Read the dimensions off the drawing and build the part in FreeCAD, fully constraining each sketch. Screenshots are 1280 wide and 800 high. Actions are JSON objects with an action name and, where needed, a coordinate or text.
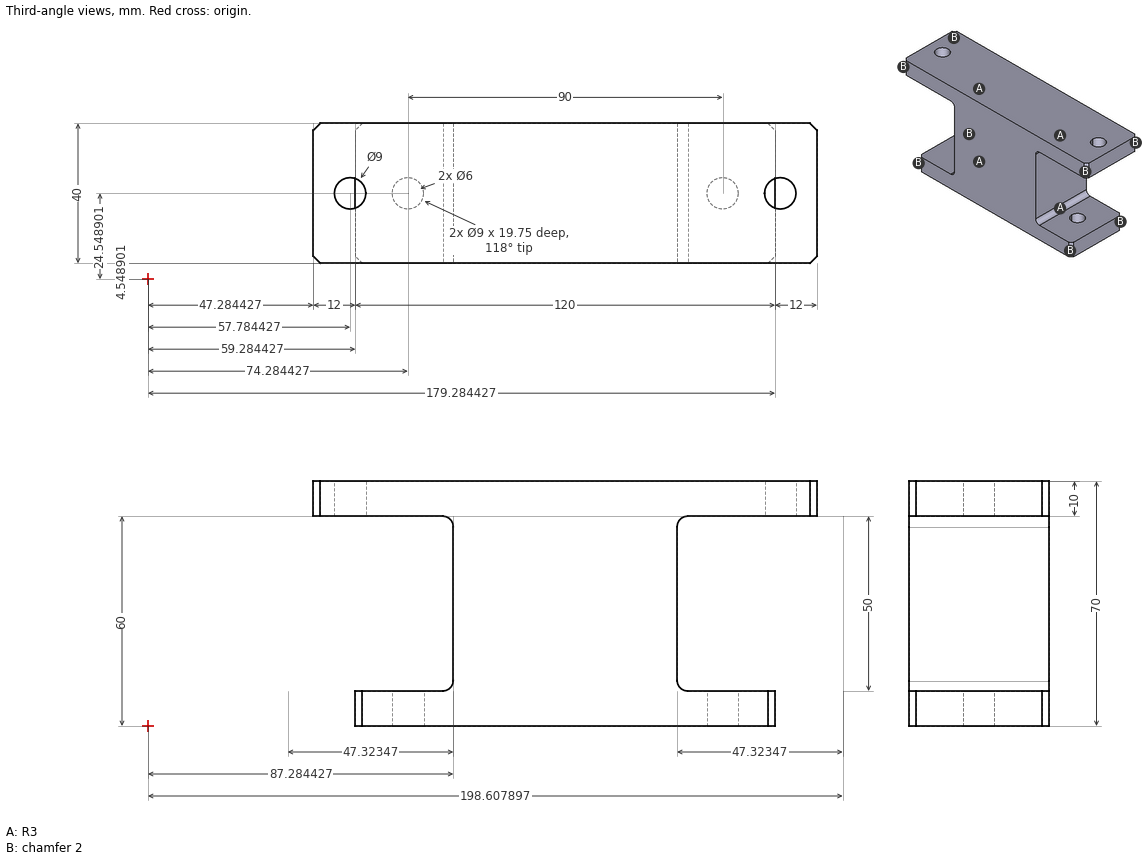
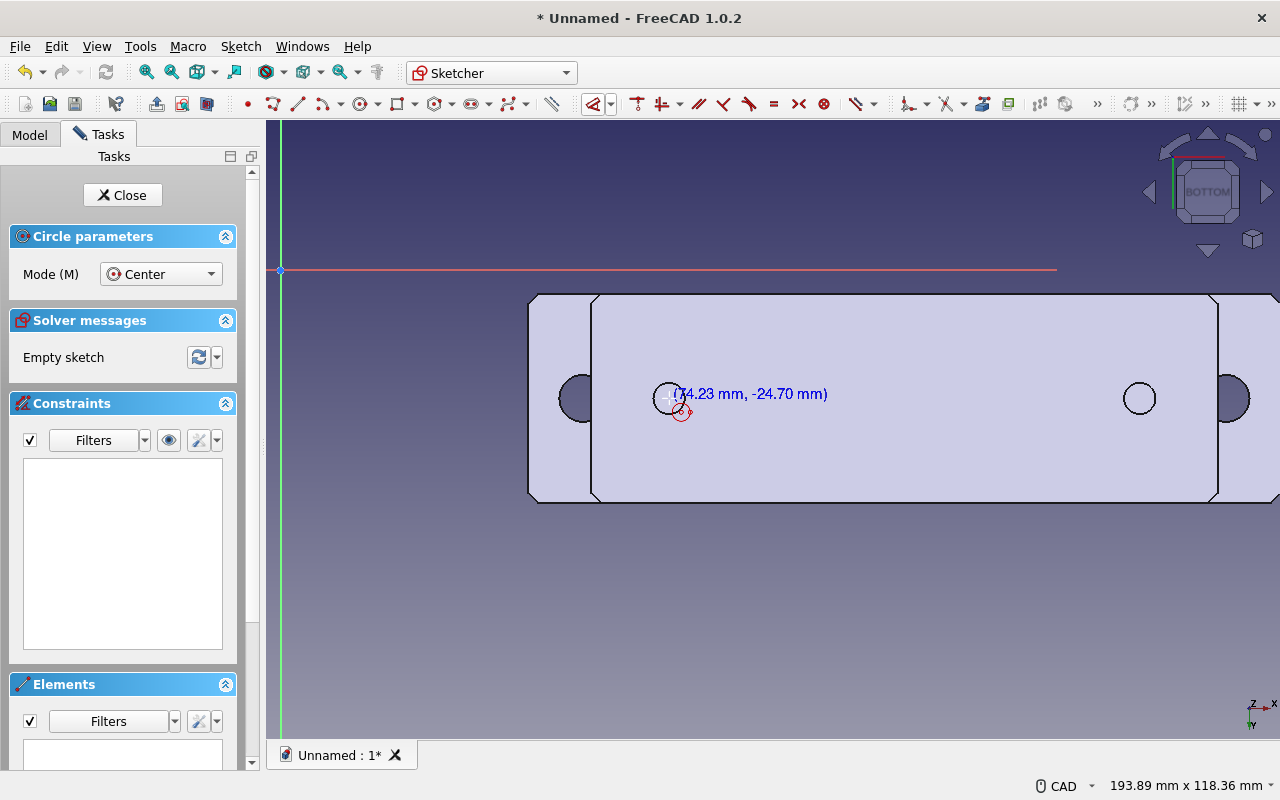
{"action": "left_click", "coordinate": [669, 398]}
{"action": "left_click", "coordinate": [686, 382]}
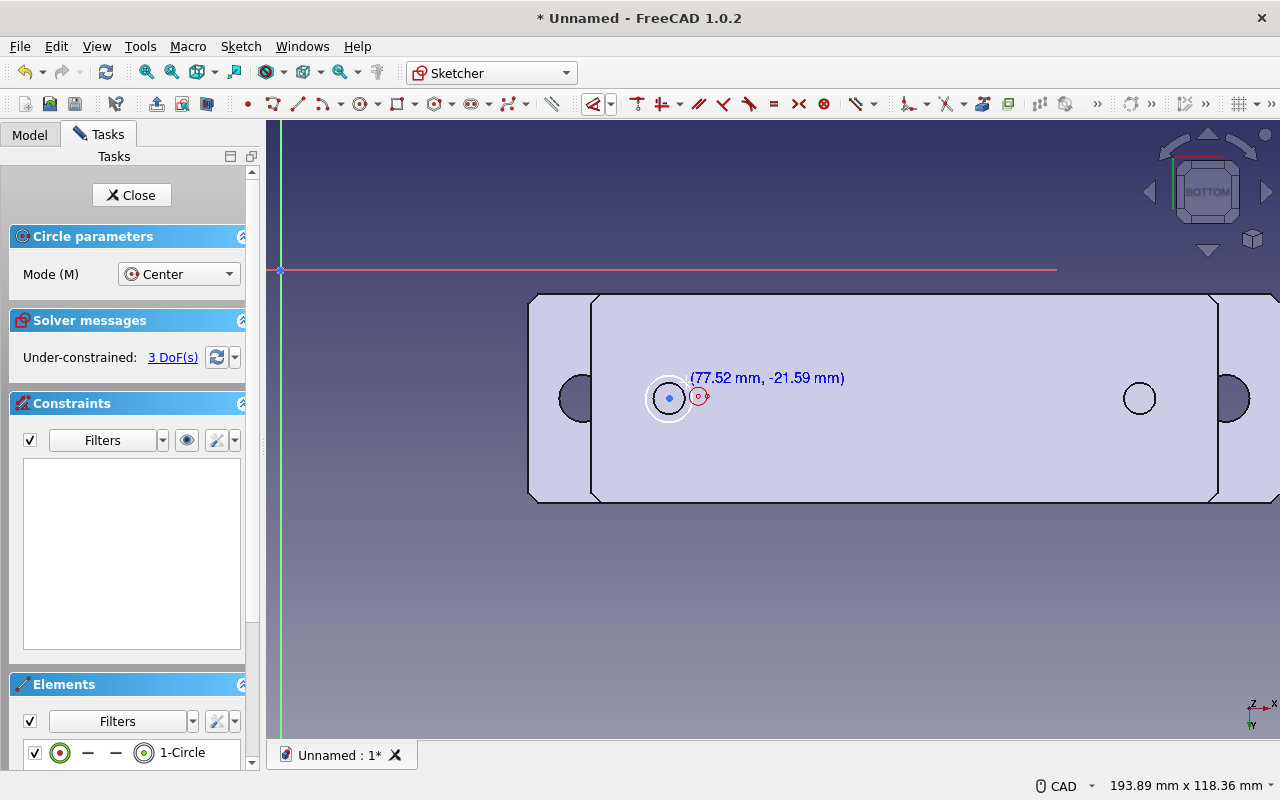
{"action": "scroll", "coordinate": [669, 599], "scroll_direction": "down", "scroll_amount": 2}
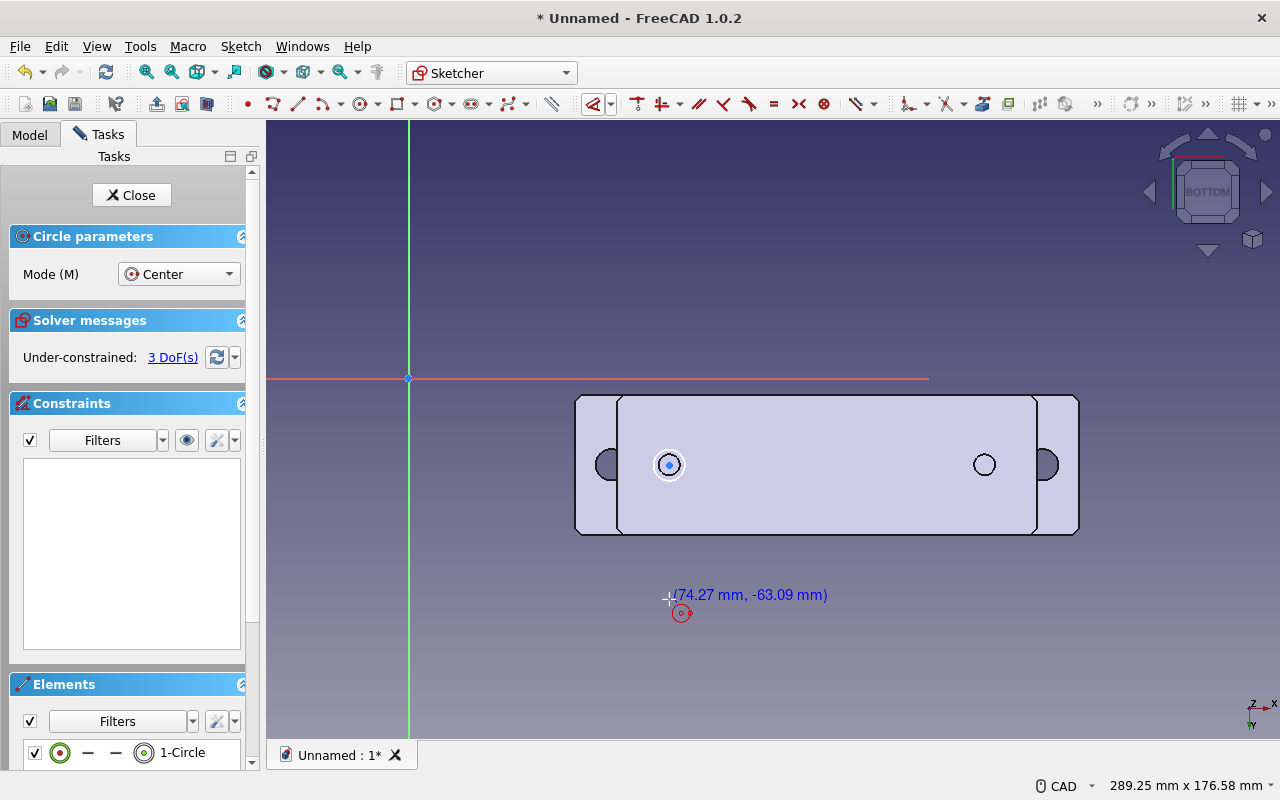
{"action": "scroll", "coordinate": [985, 465], "scroll_direction": "up", "scroll_amount": 2}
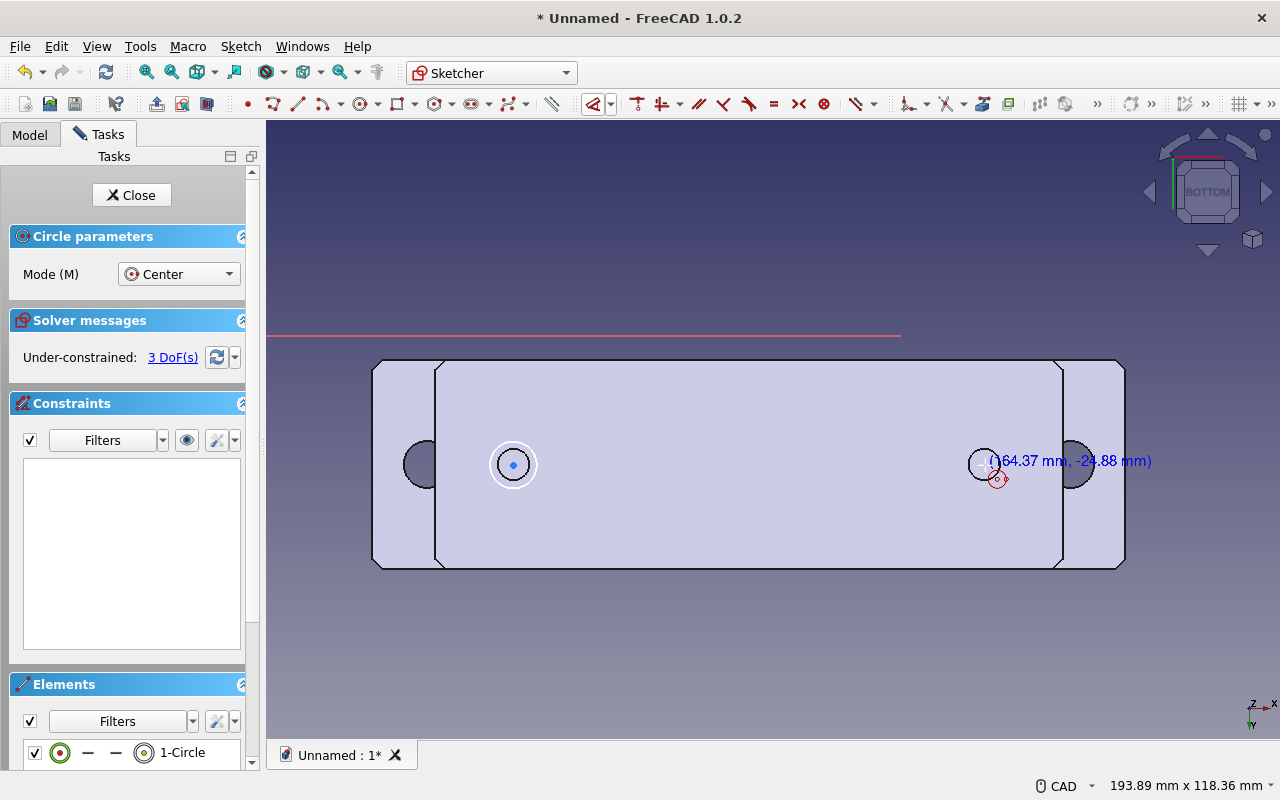
{"action": "left_click", "coordinate": [984, 464]}
{"action": "left_click", "coordinate": [1001, 448]}
{"action": "key", "text": "Escape"}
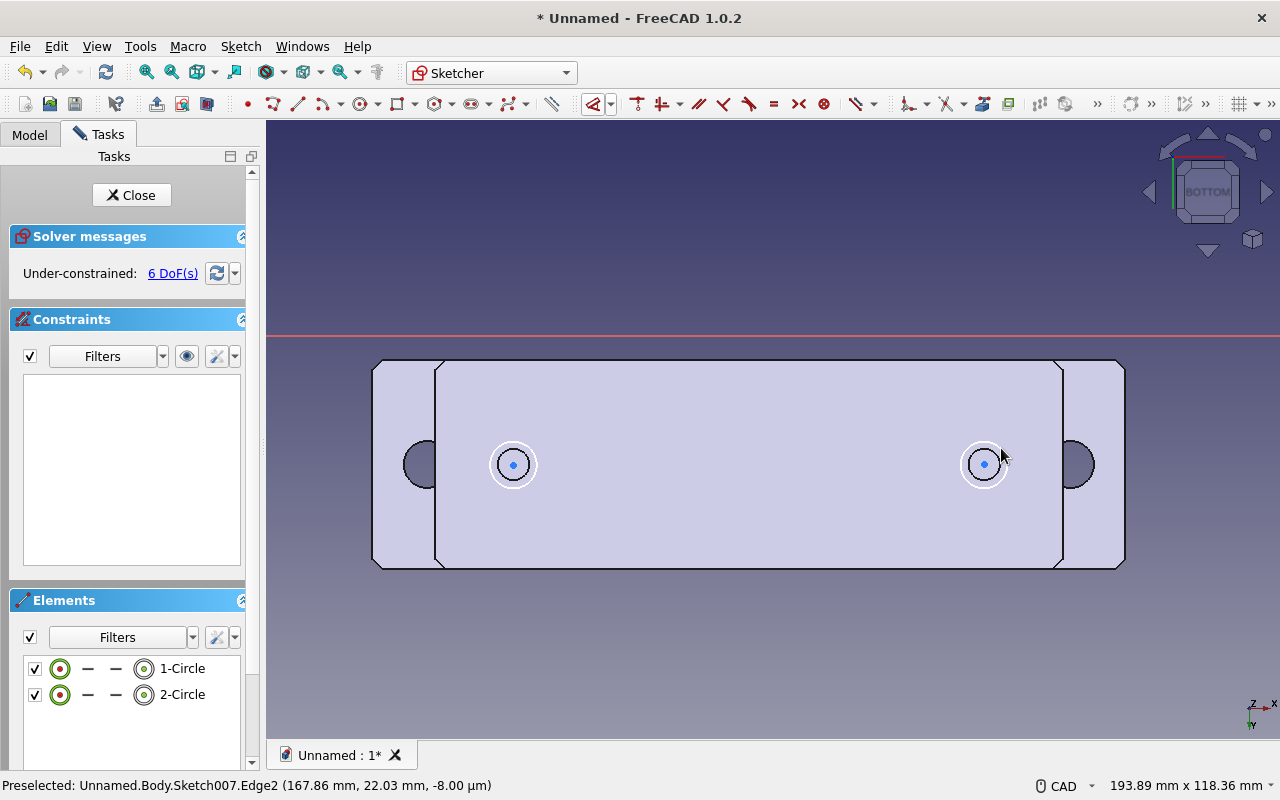
{"action": "left_click", "coordinate": [530, 448]}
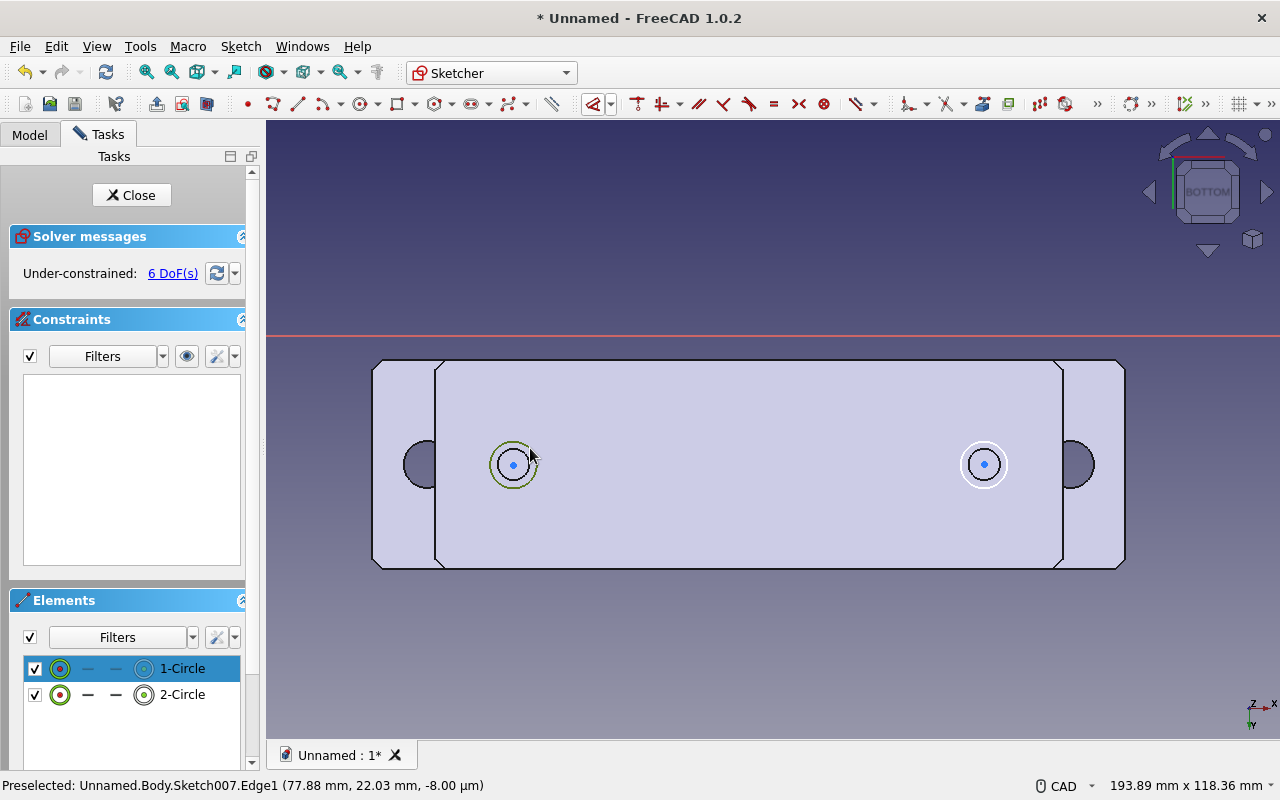
{"action": "left_click", "coordinate": [1000, 448]}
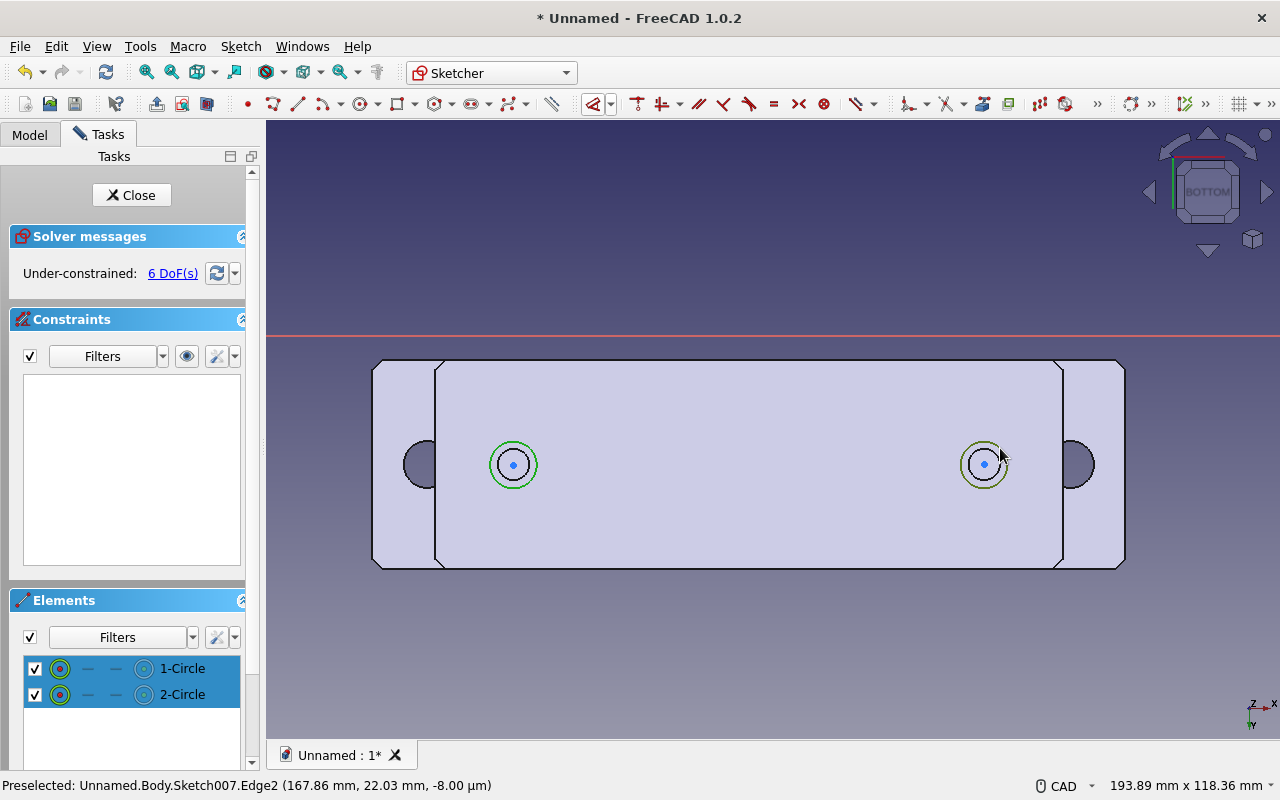
{"action": "key", "text": "e"}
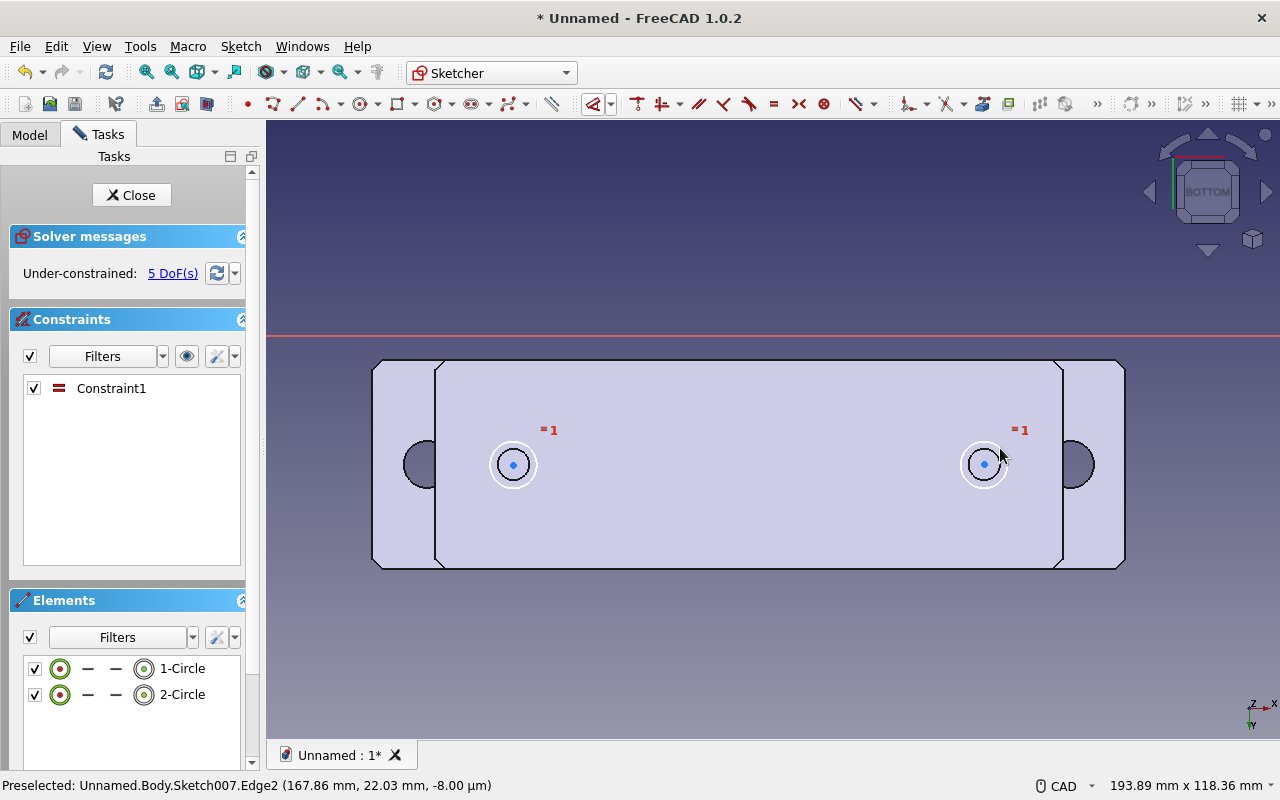
{"action": "left_click", "coordinate": [513, 465]}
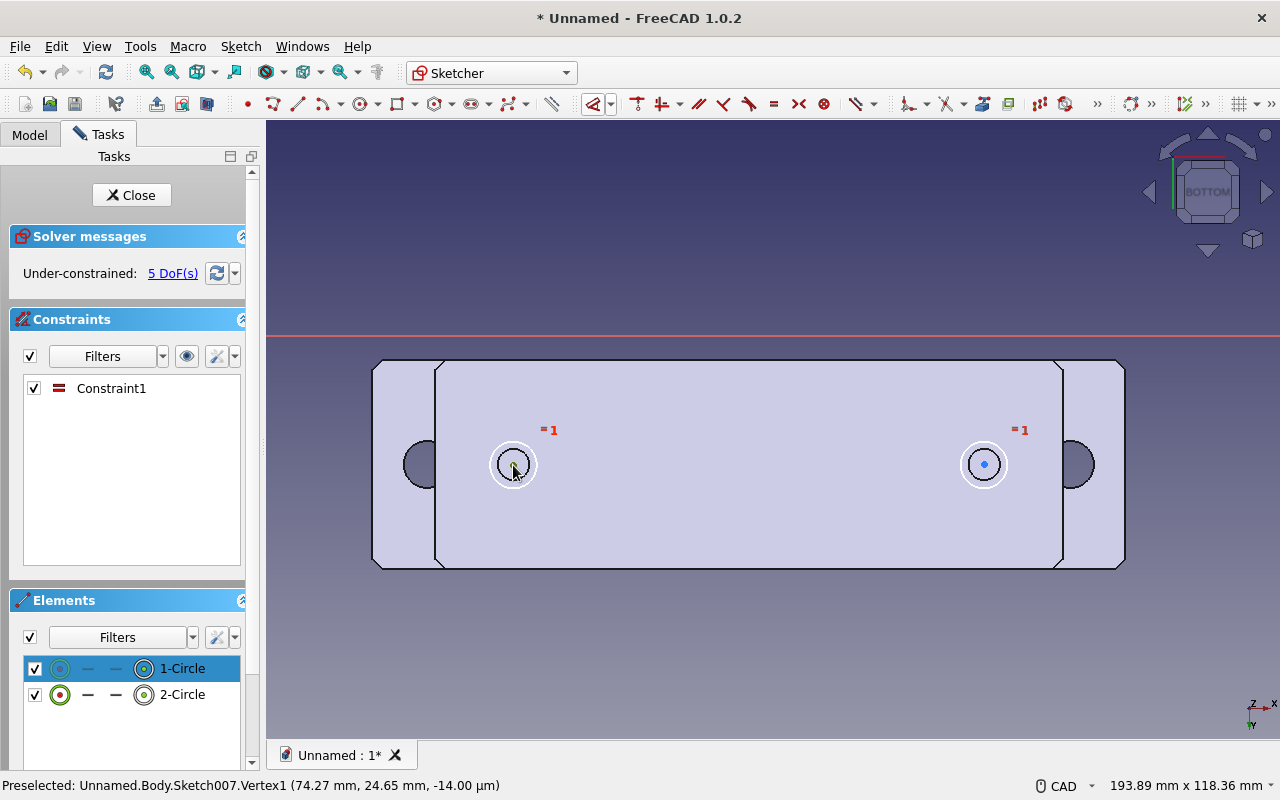
{"action": "left_click", "coordinate": [984, 465]}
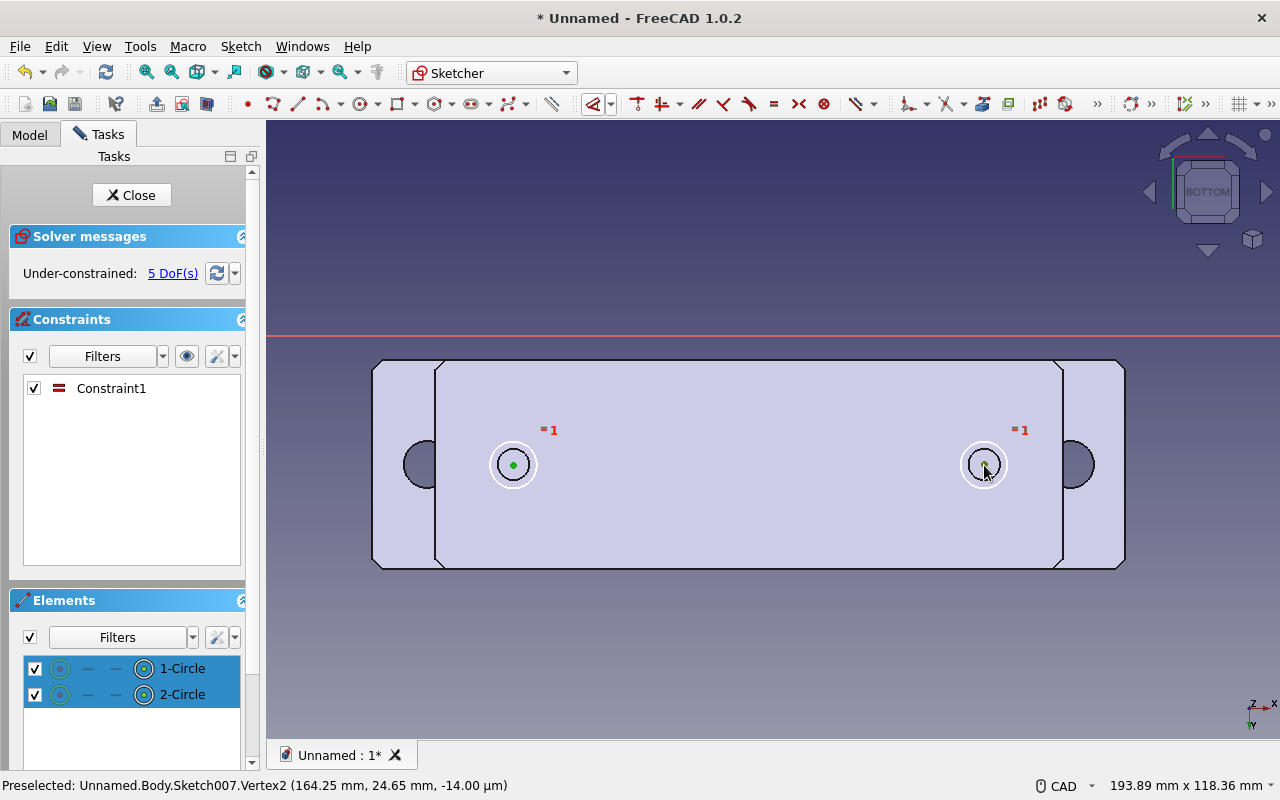
{"action": "left_click", "coordinate": [680, 104]}